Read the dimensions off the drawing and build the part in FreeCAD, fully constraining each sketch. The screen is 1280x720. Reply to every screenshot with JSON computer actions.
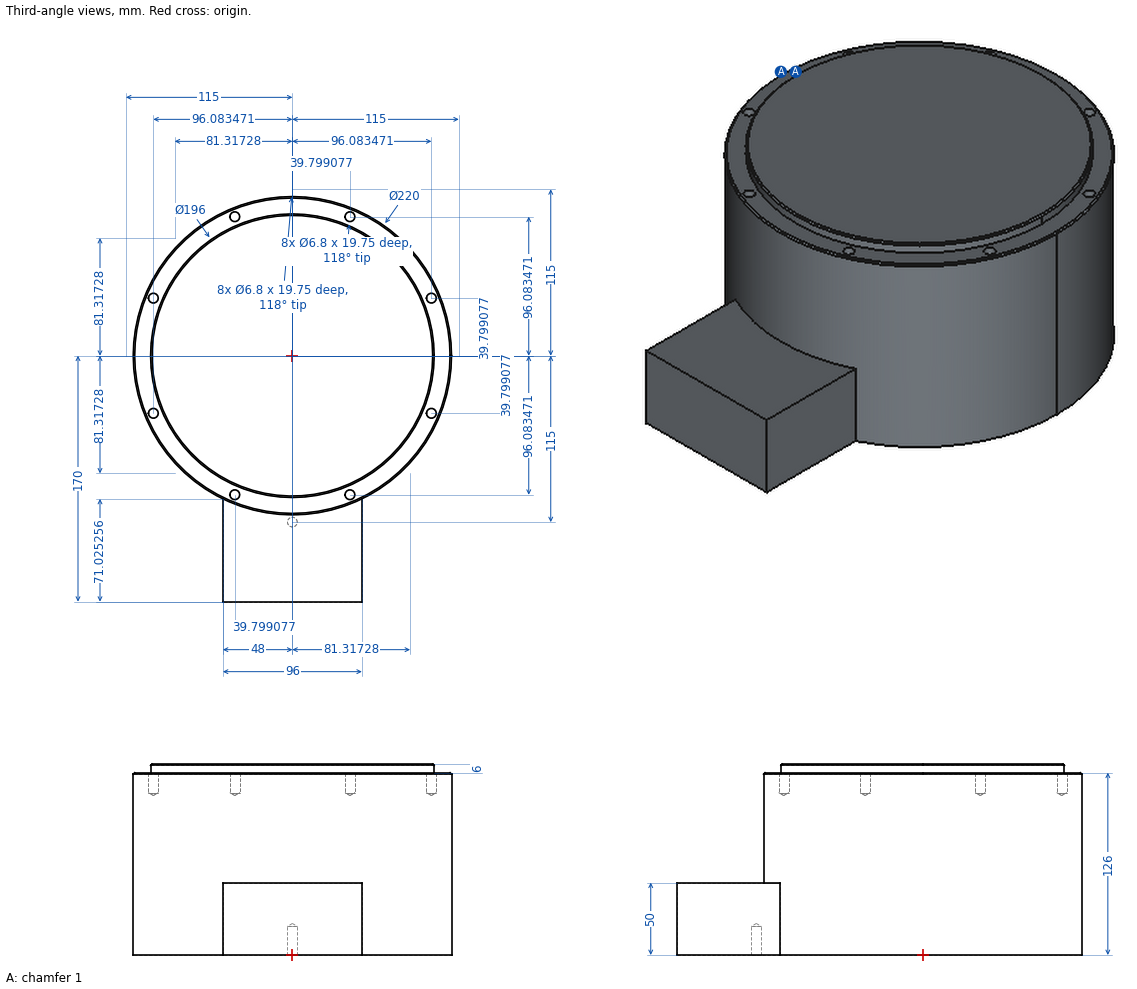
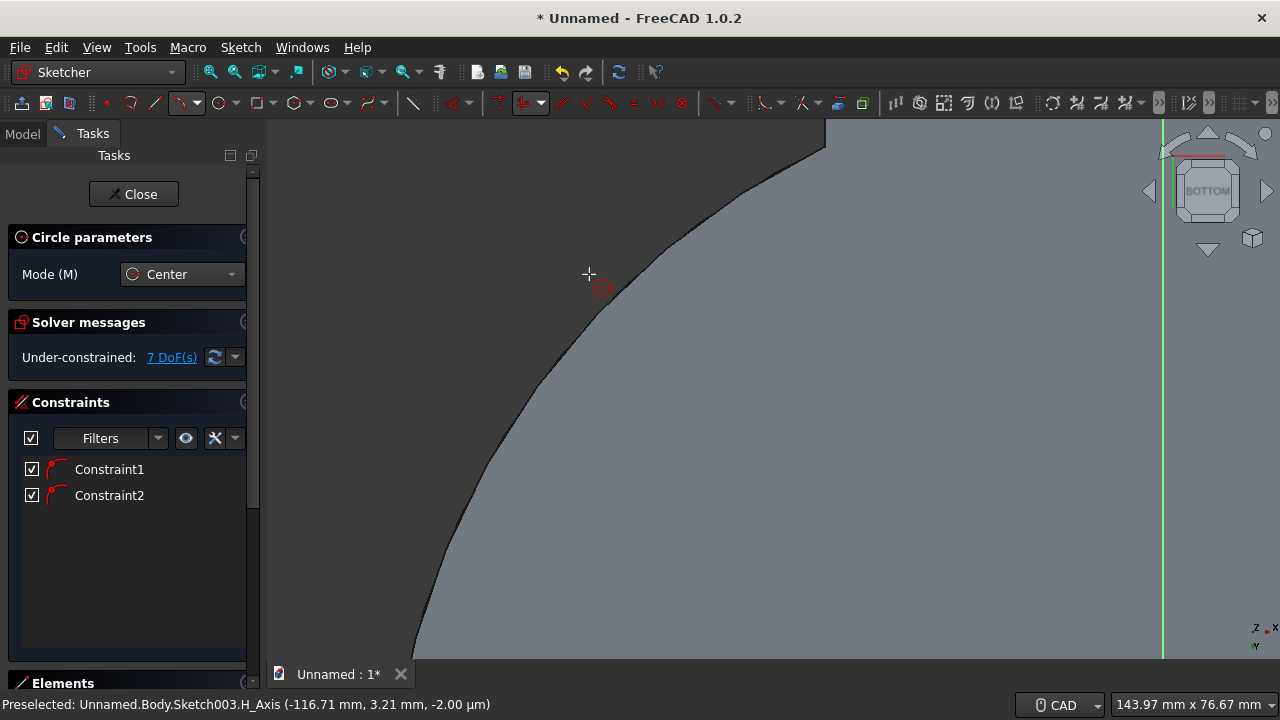
{"action": "scroll", "coordinate": [589, 274], "scroll_direction": "down", "scroll_amount": 8}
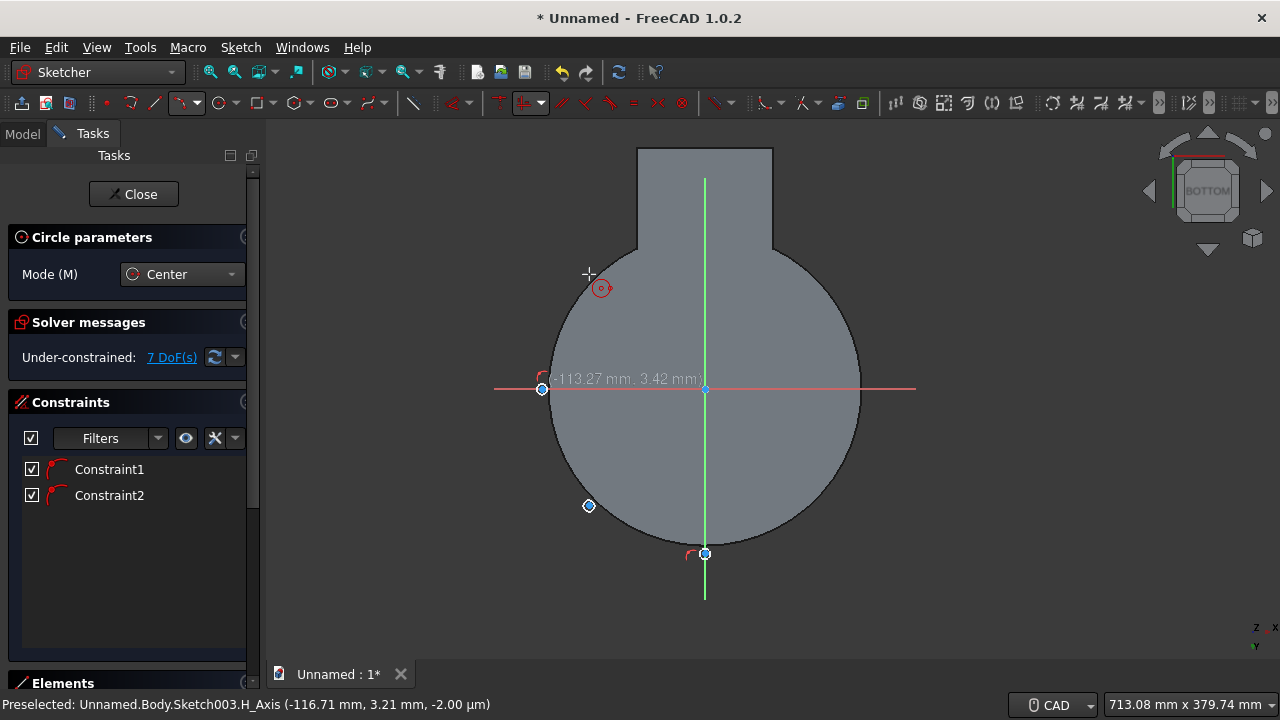
{"action": "left_click", "coordinate": [589, 274]}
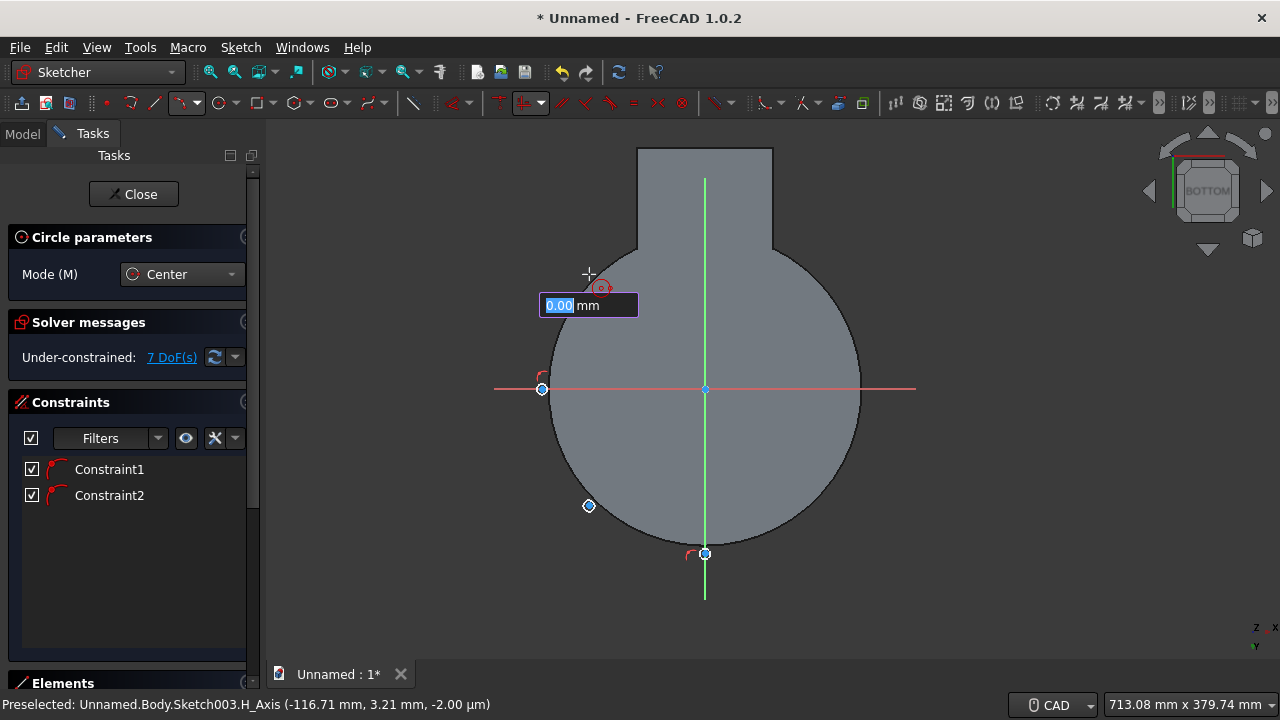
{"action": "scroll", "coordinate": [593, 270], "scroll_direction": "up", "scroll_amount": 6}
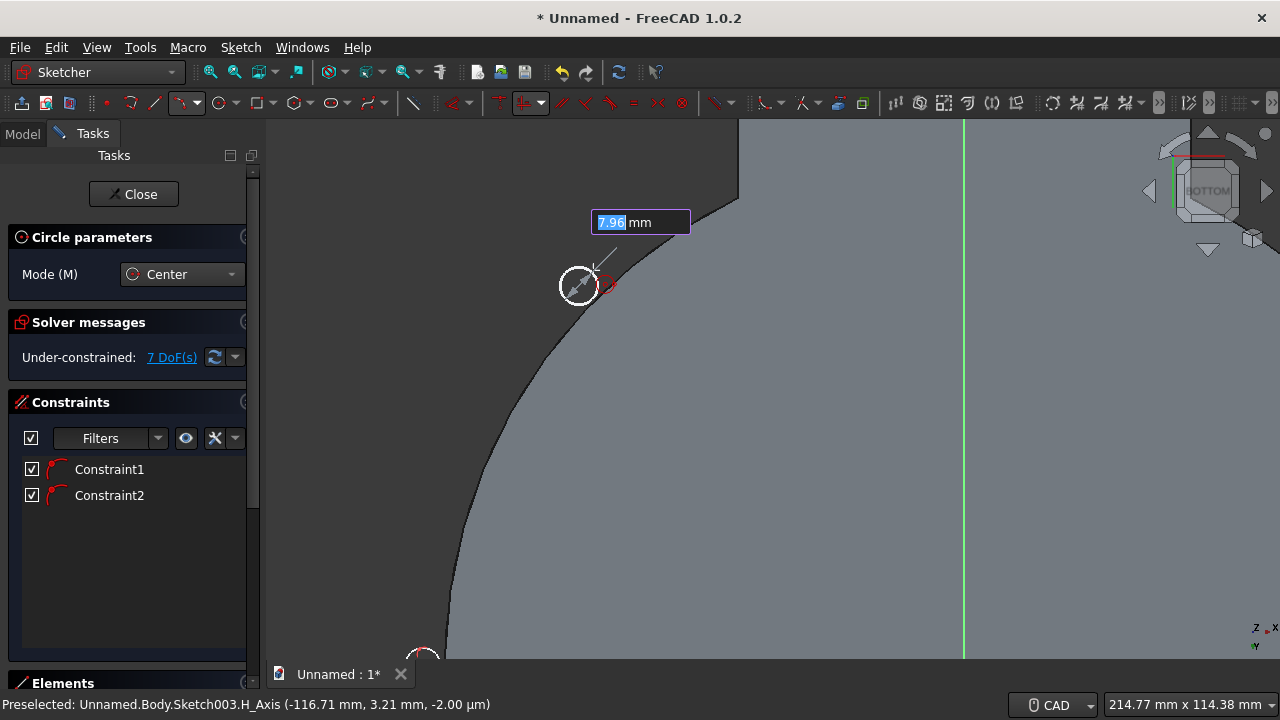
{"action": "left_click", "coordinate": [592, 270]}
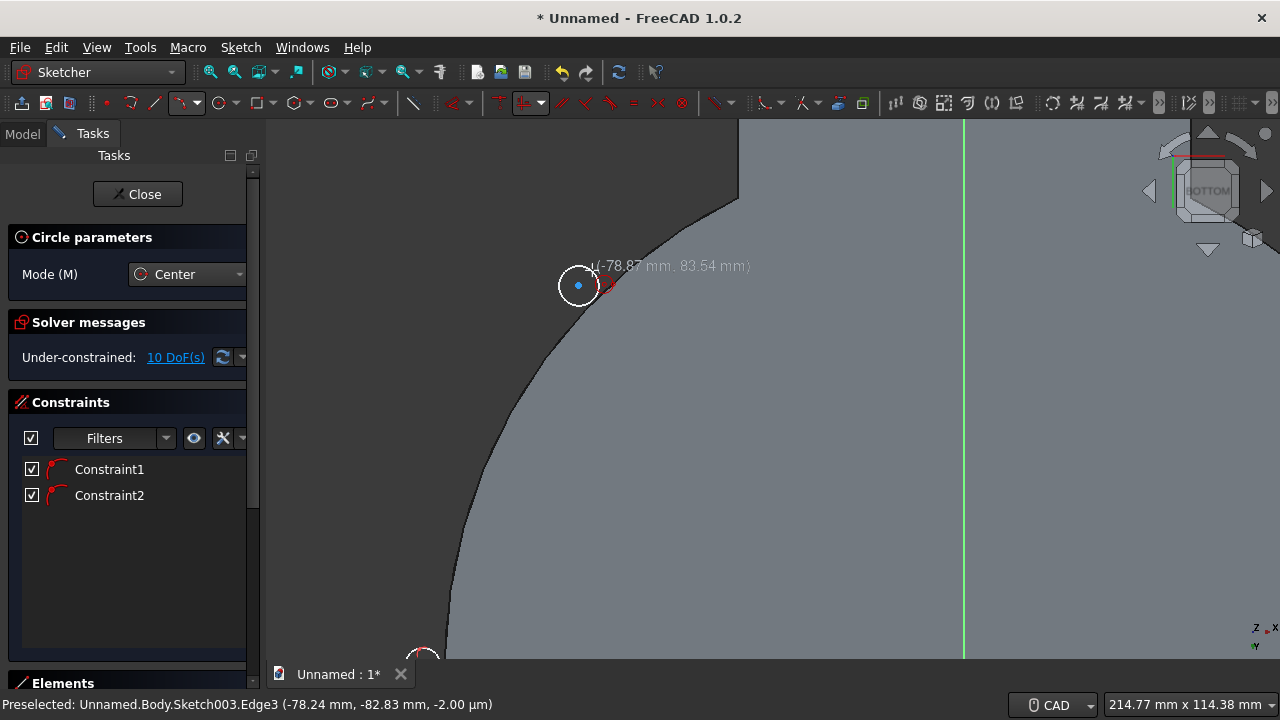
{"action": "scroll", "coordinate": [593, 270], "scroll_direction": "down", "scroll_amount": 6}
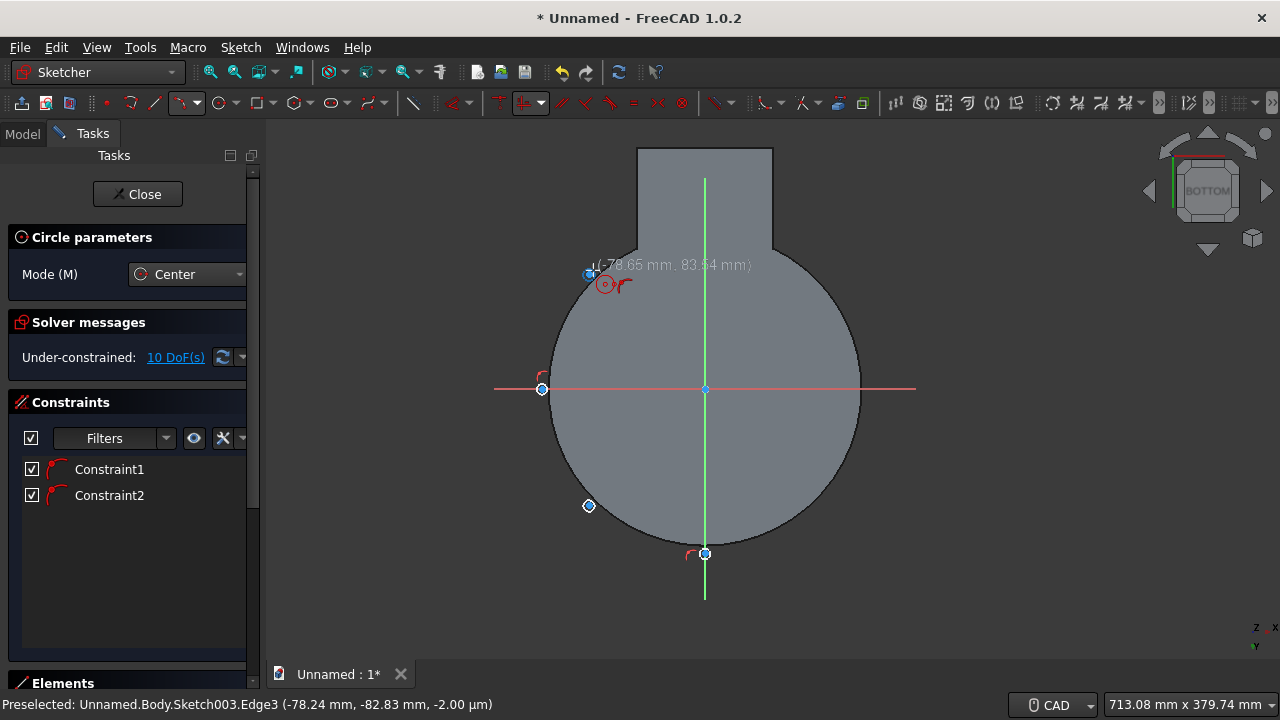
{"action": "scroll", "coordinate": [705, 226], "scroll_direction": "up", "scroll_amount": 8}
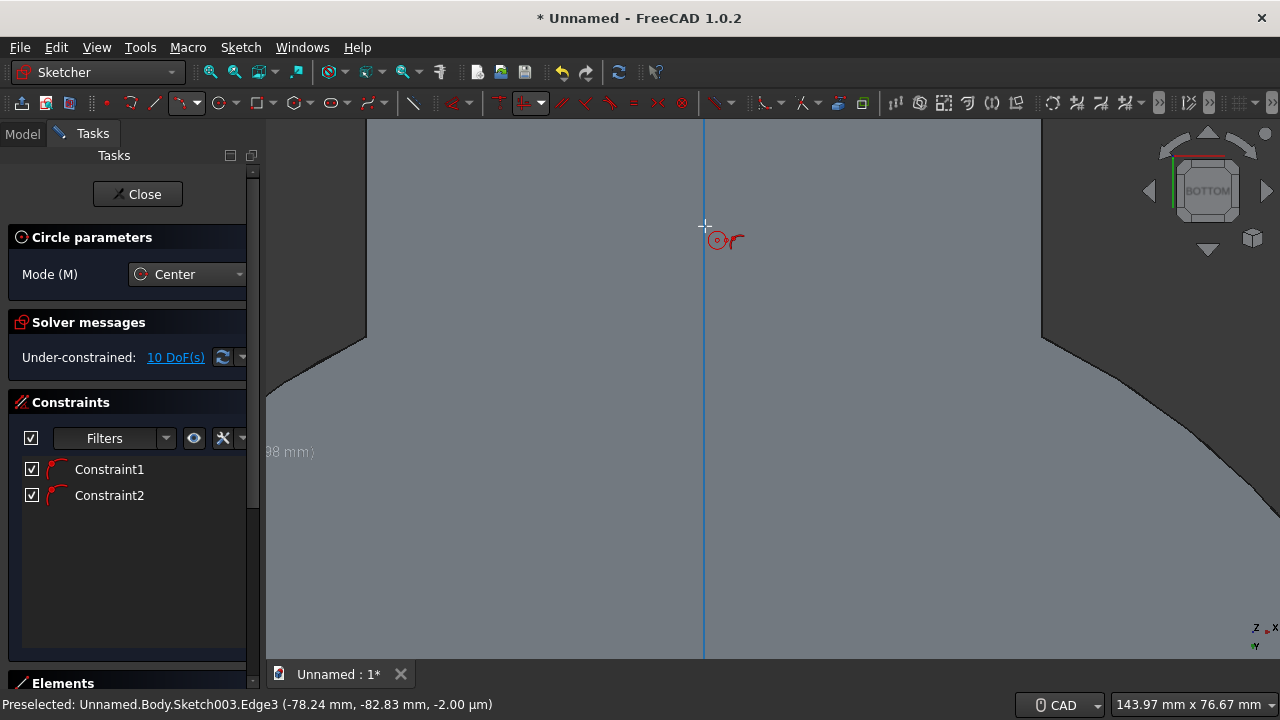
{"action": "scroll", "coordinate": [705, 226], "scroll_direction": "down", "scroll_amount": 8}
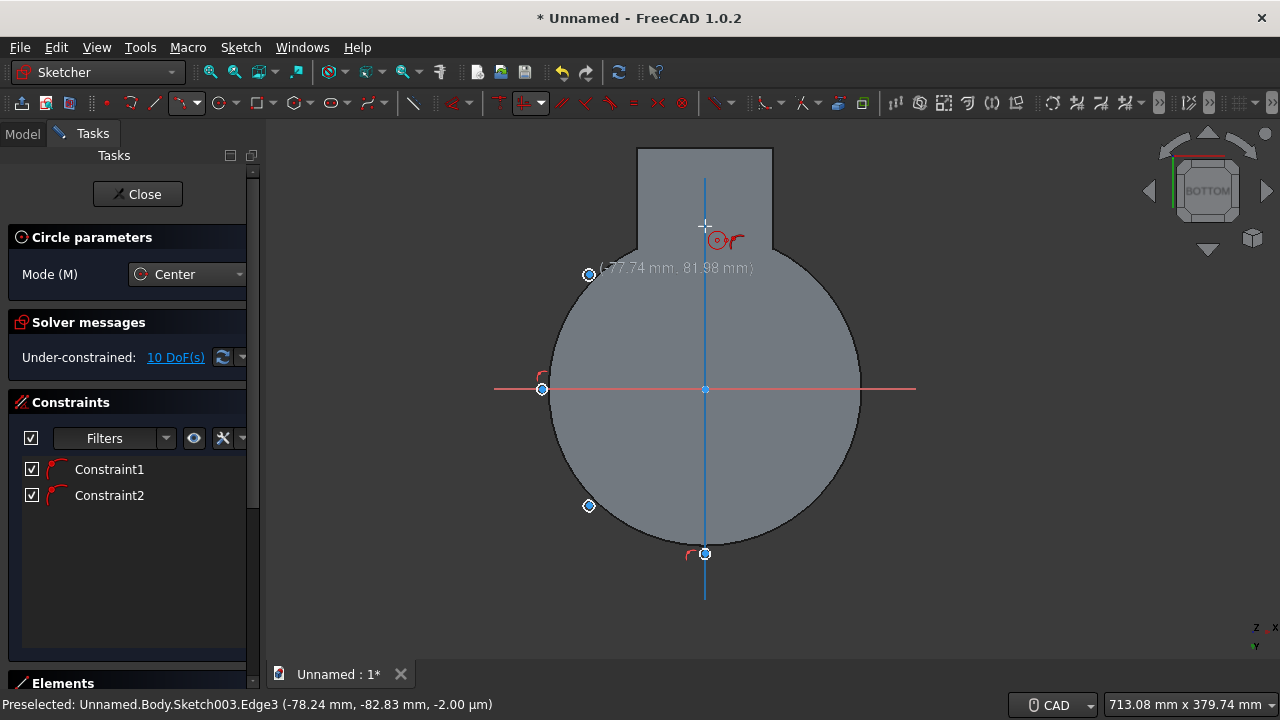
{"action": "left_click", "coordinate": [705, 226]}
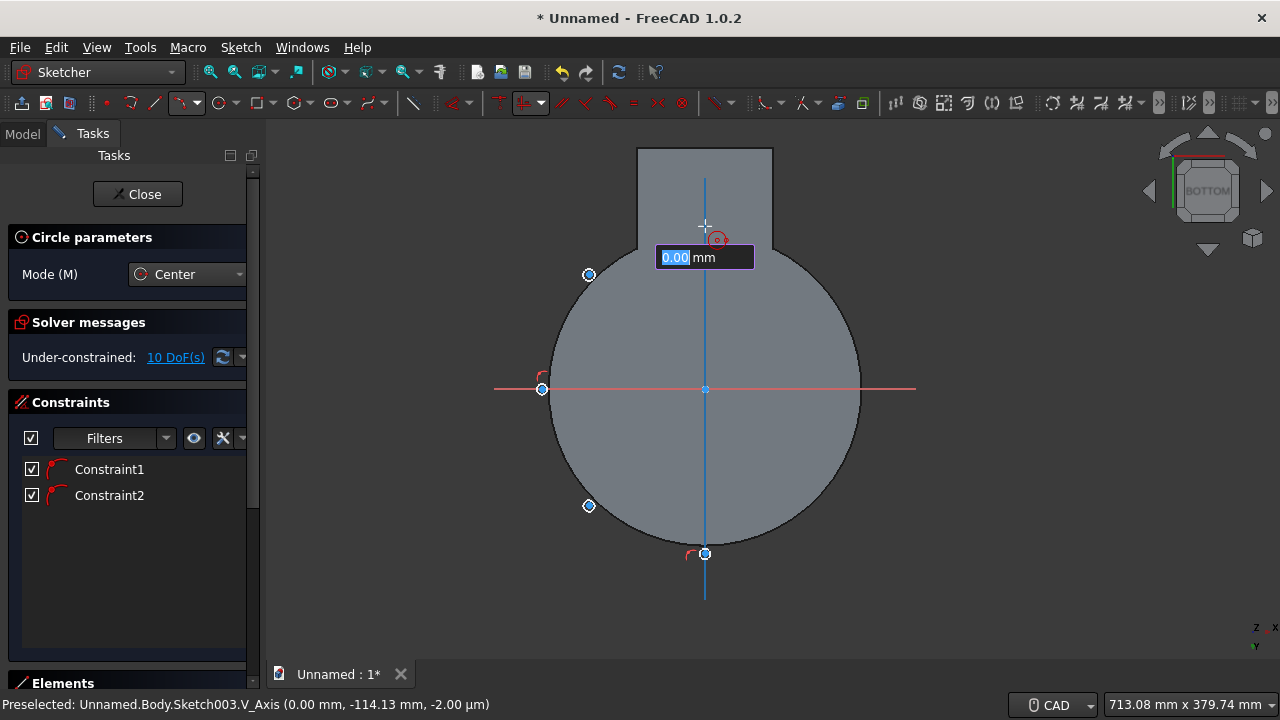
{"action": "scroll", "coordinate": [710, 224], "scroll_direction": "up", "scroll_amount": 7}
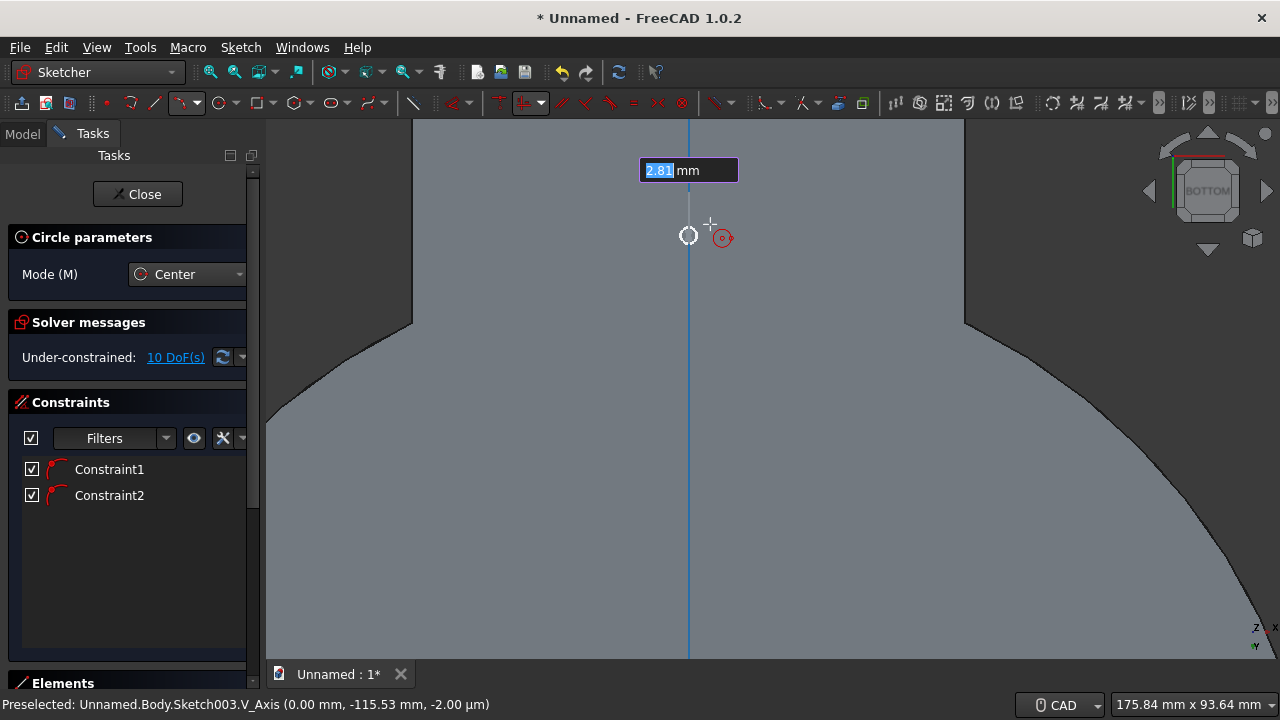
{"action": "left_click", "coordinate": [707, 224]}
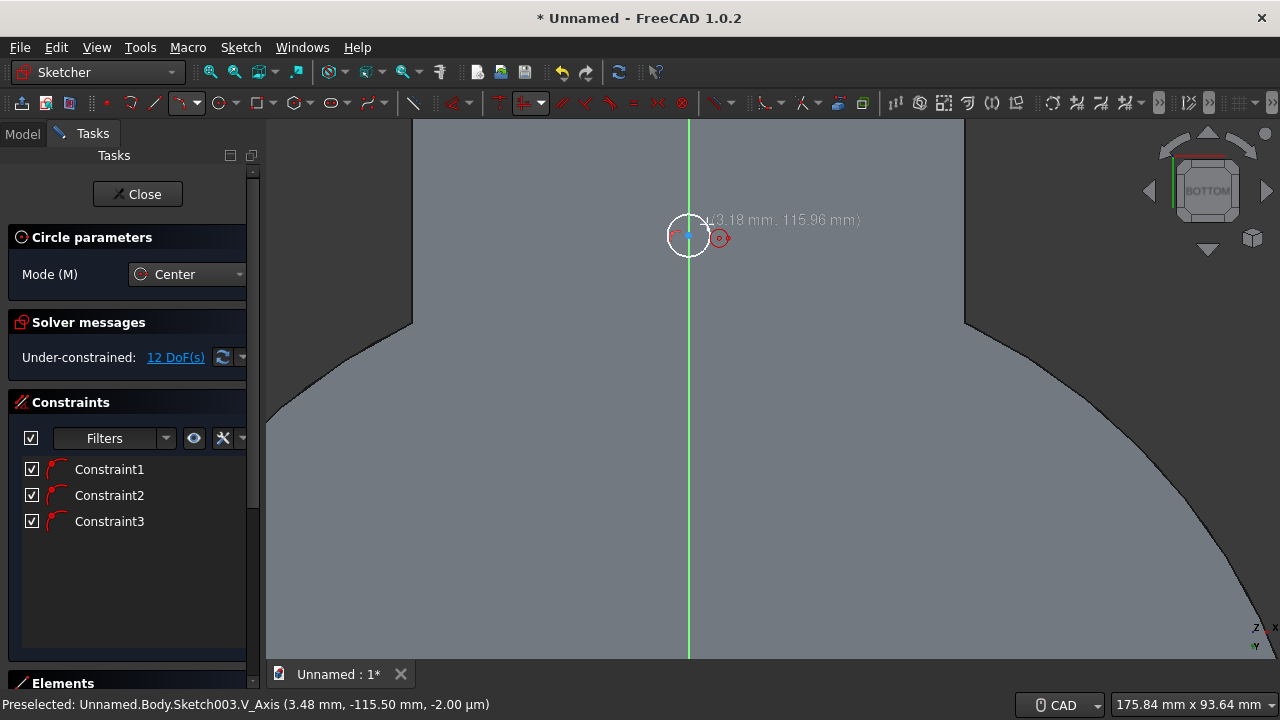
{"action": "scroll", "coordinate": [710, 224], "scroll_direction": "down", "scroll_amount": 7}